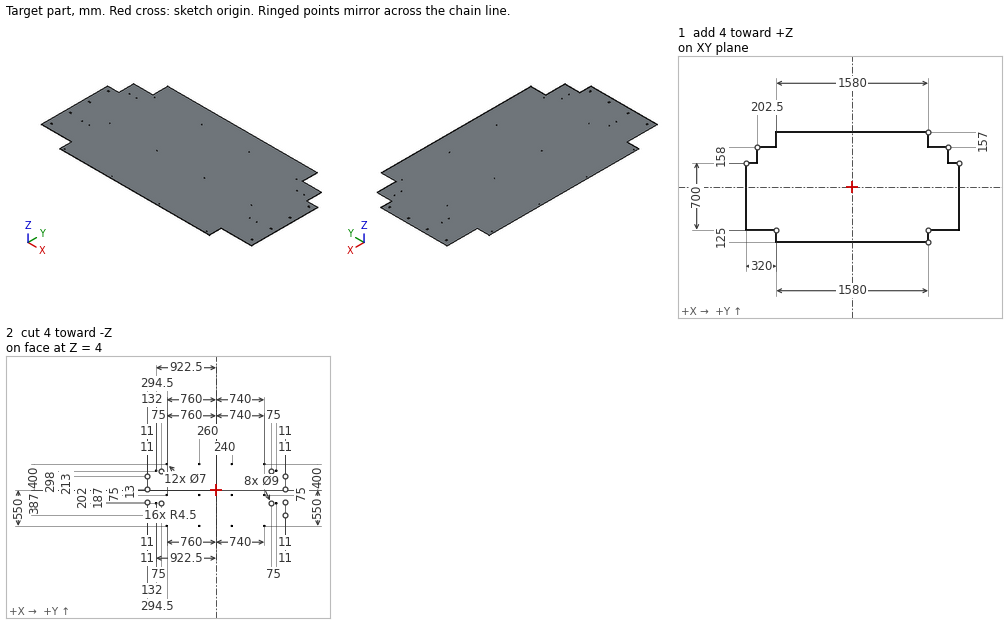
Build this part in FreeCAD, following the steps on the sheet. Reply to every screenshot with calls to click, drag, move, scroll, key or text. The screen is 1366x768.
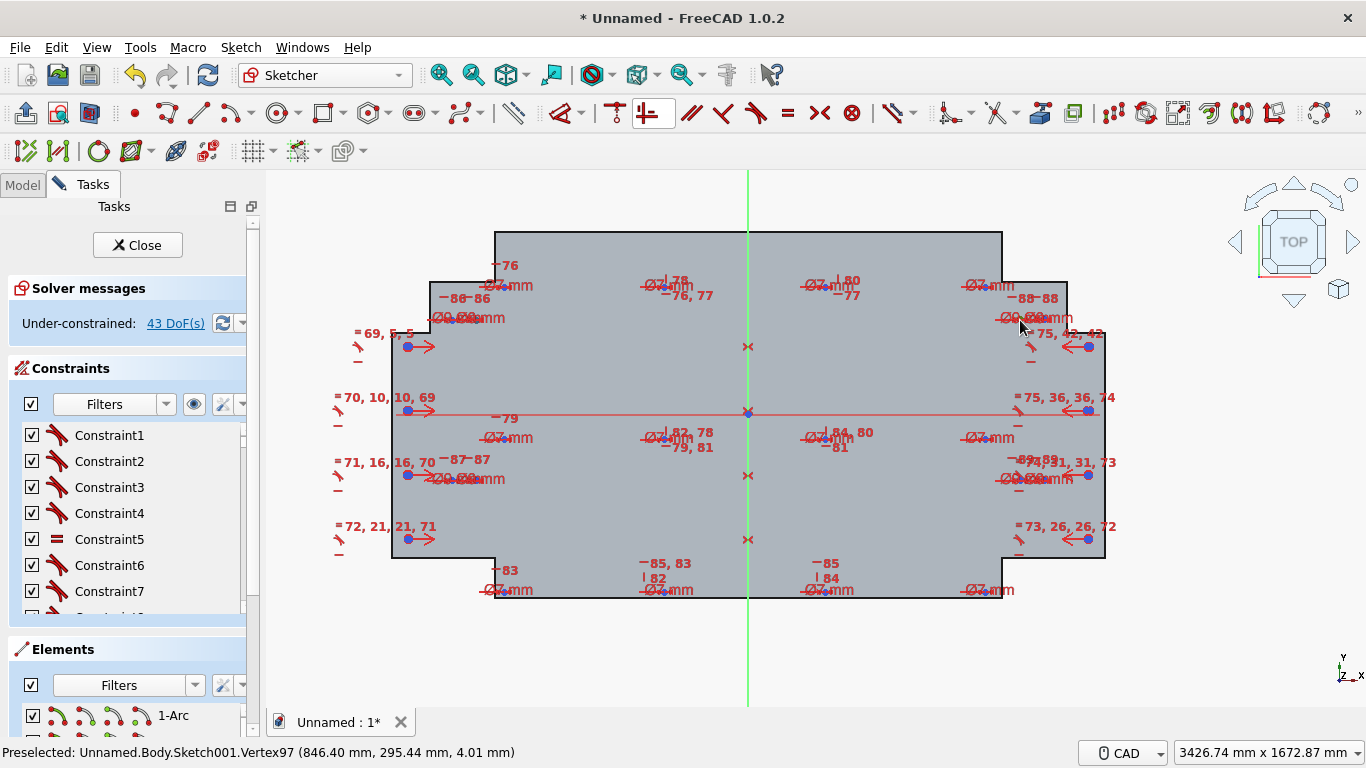
click(748, 645)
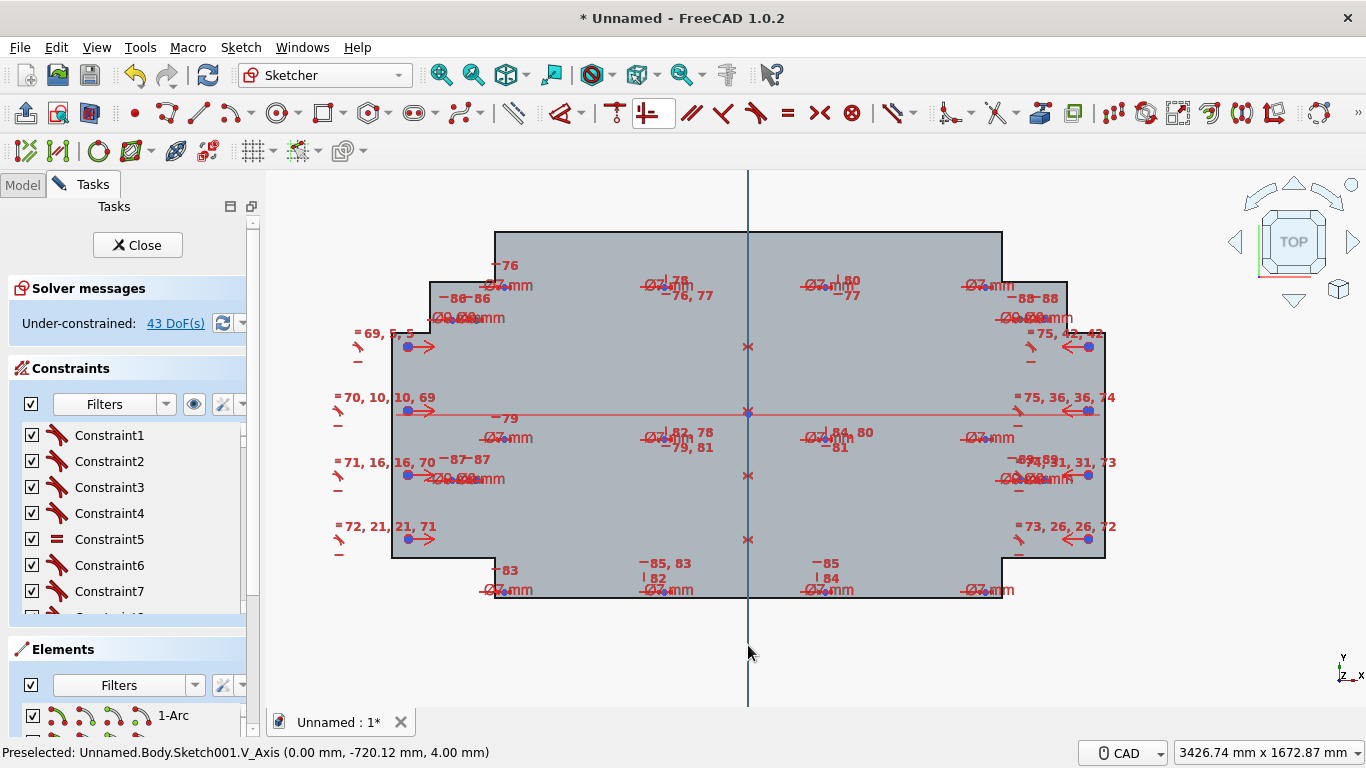
click(820, 114)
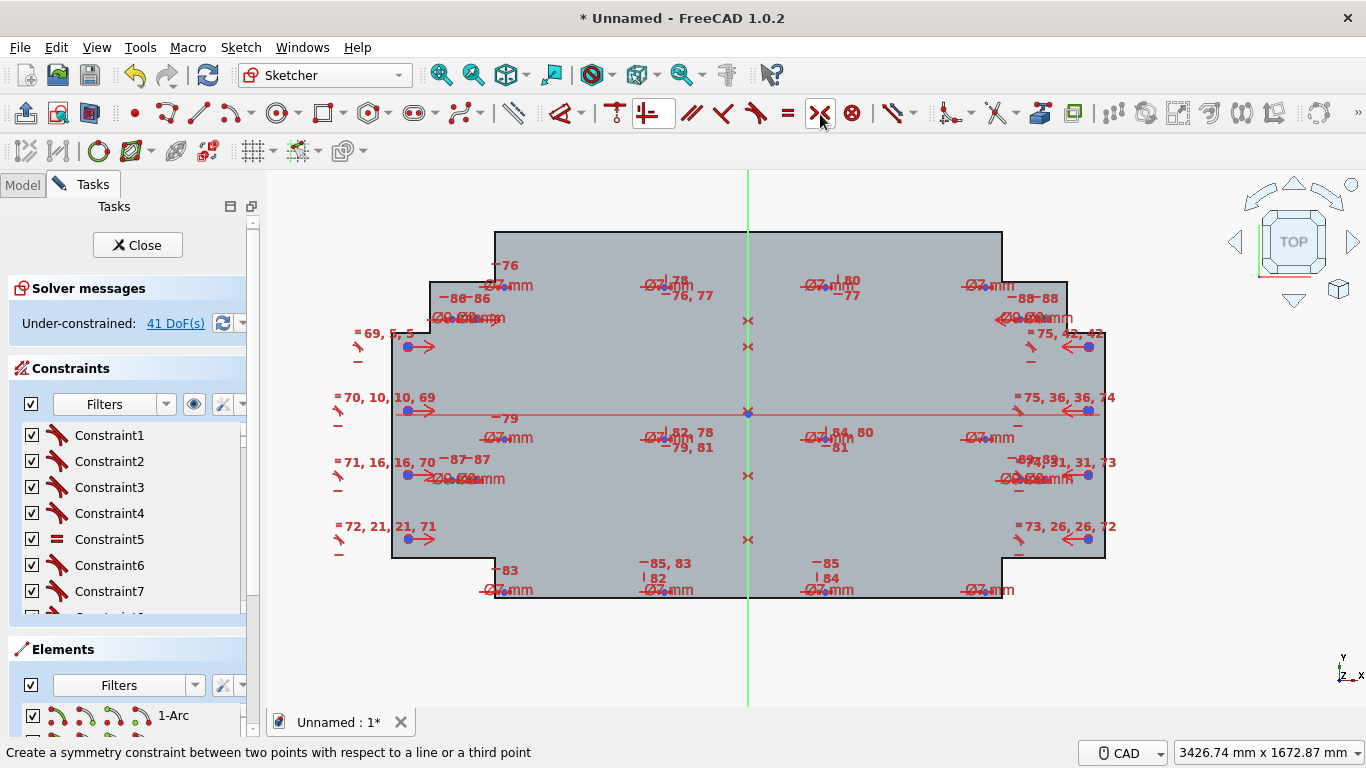
click(476, 481)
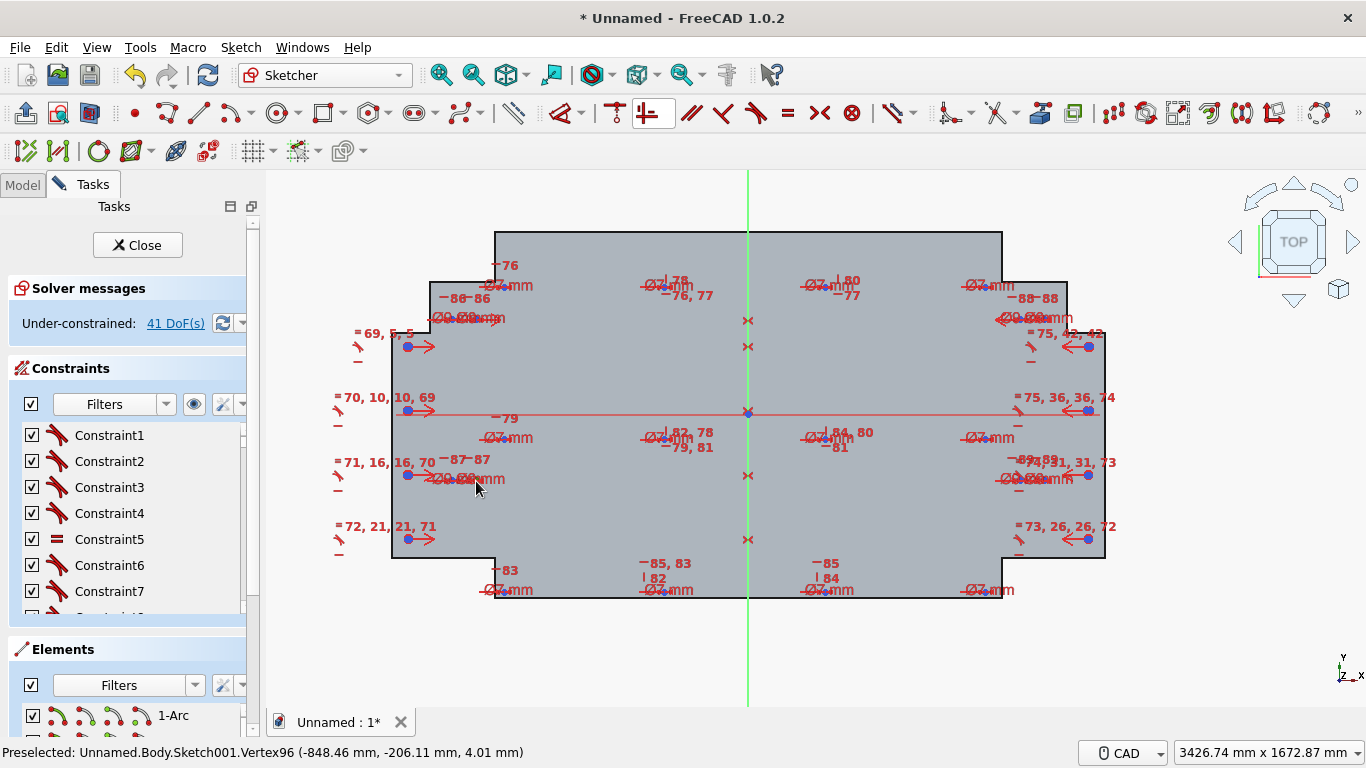
click(1020, 481)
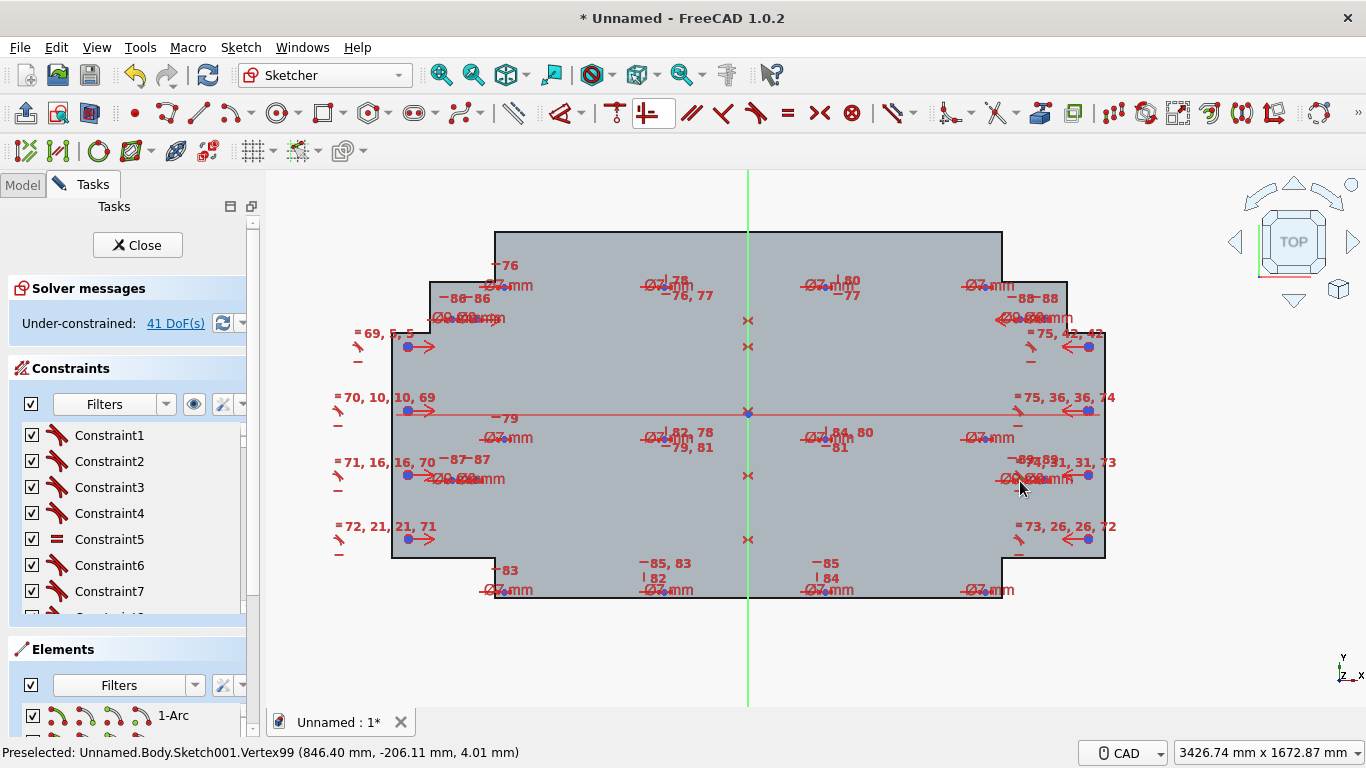
click(748, 645)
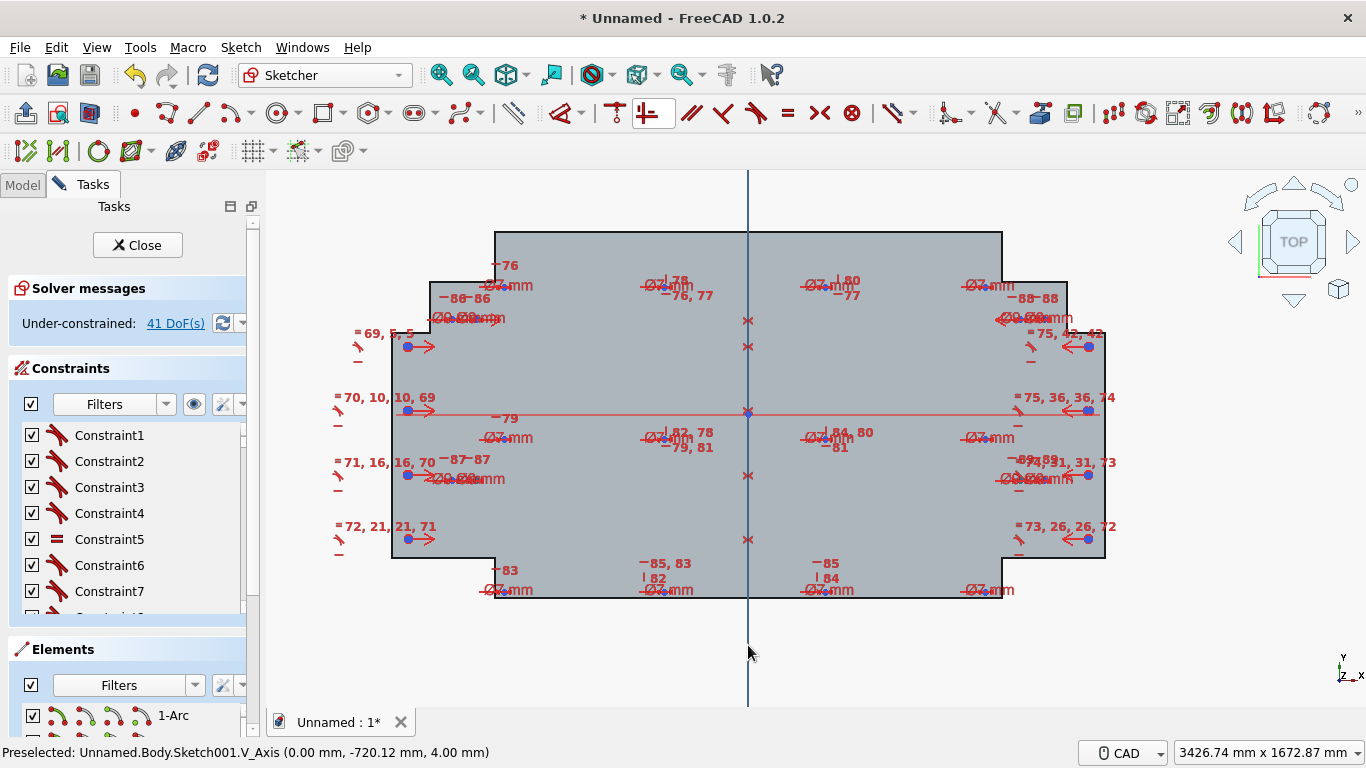
click(820, 114)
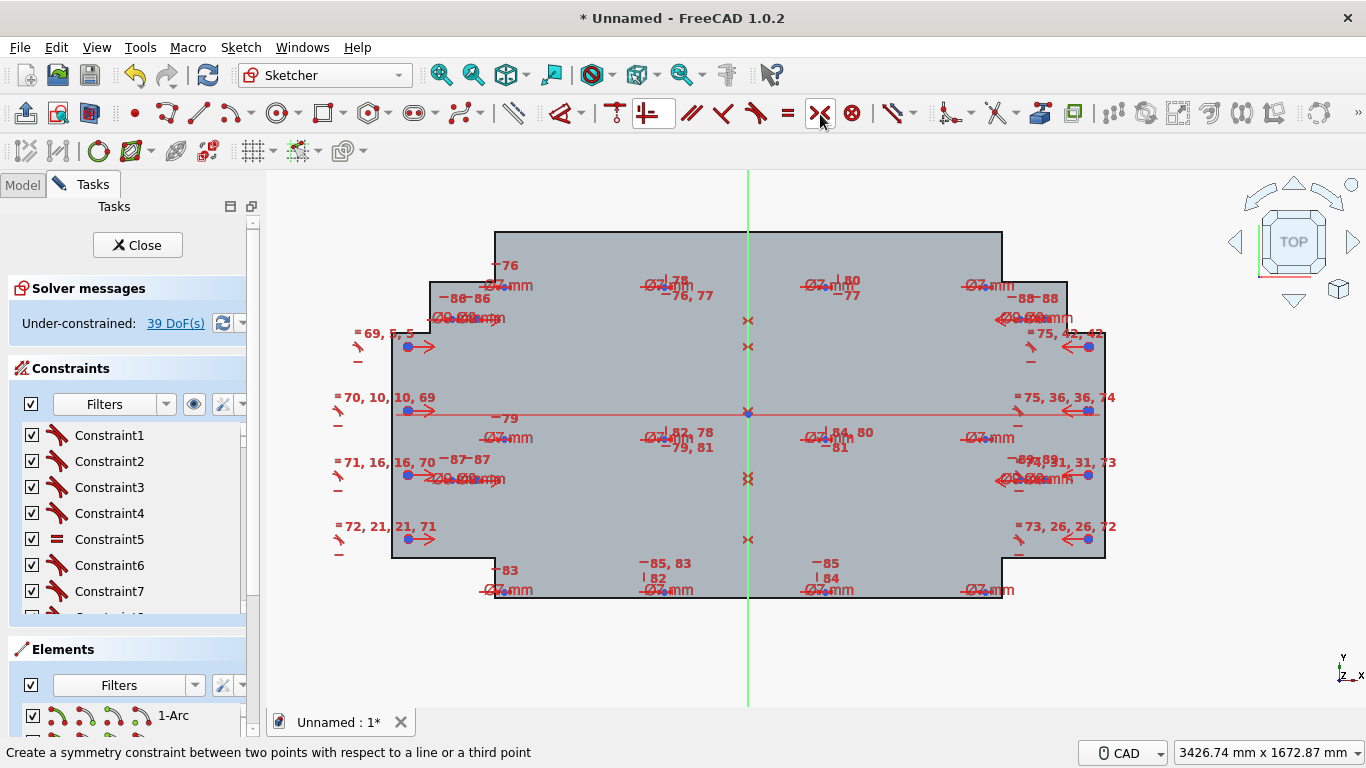
click(560, 114)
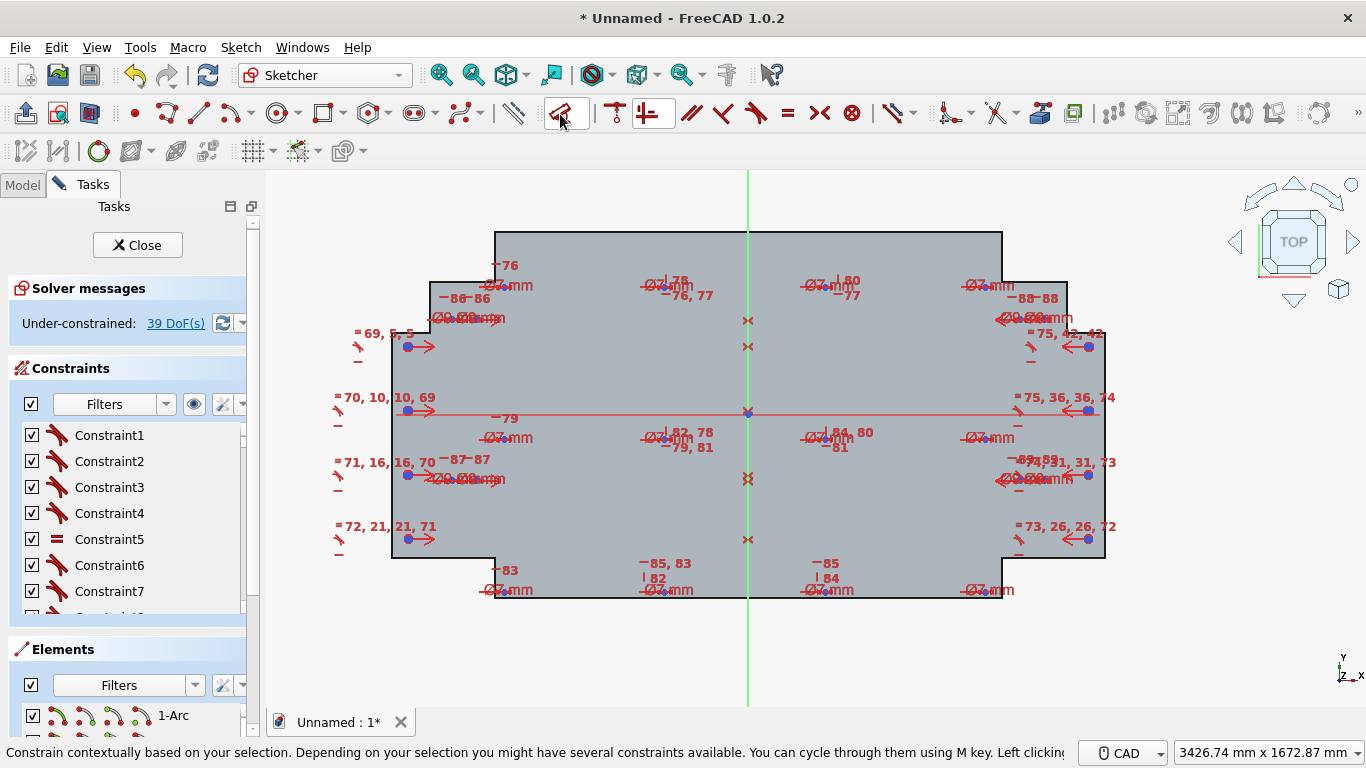
scroll(405, 347, up, 17)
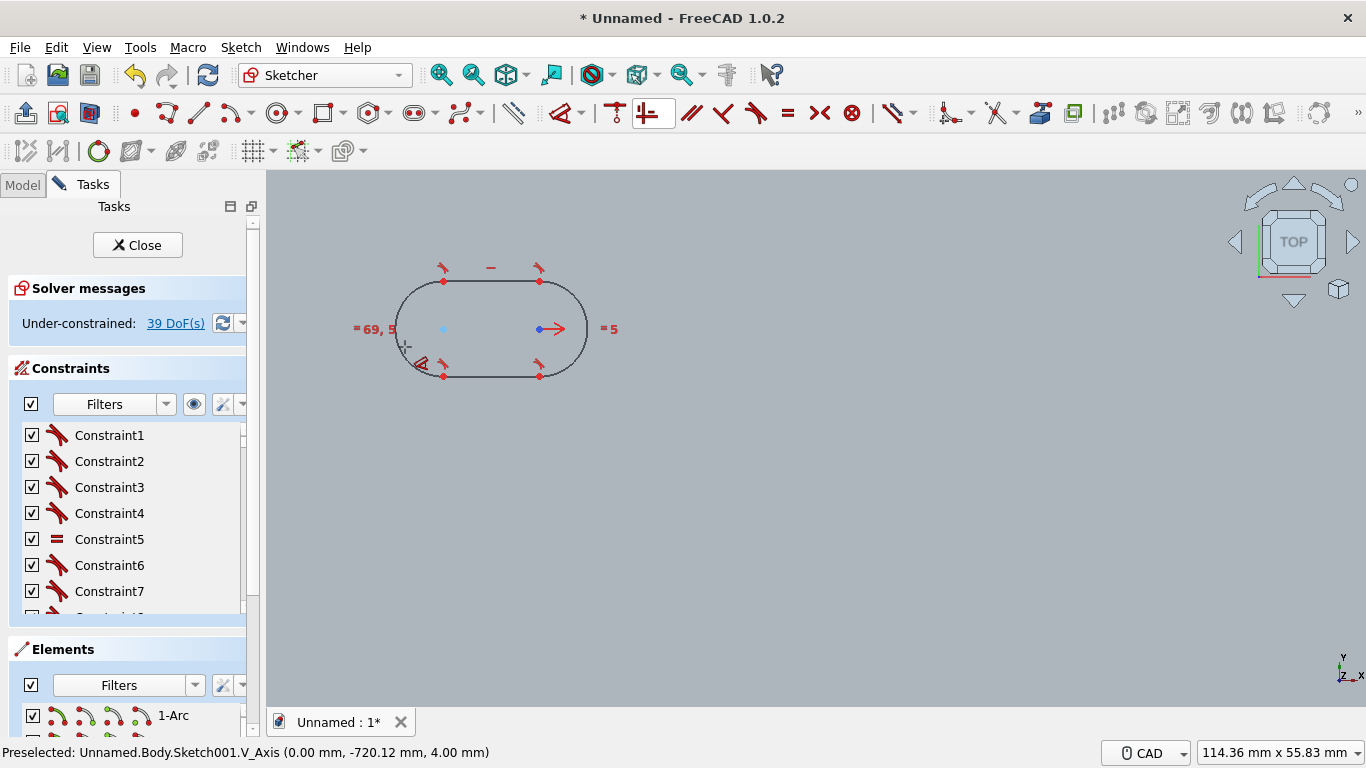
click(395, 329)
click(363, 329)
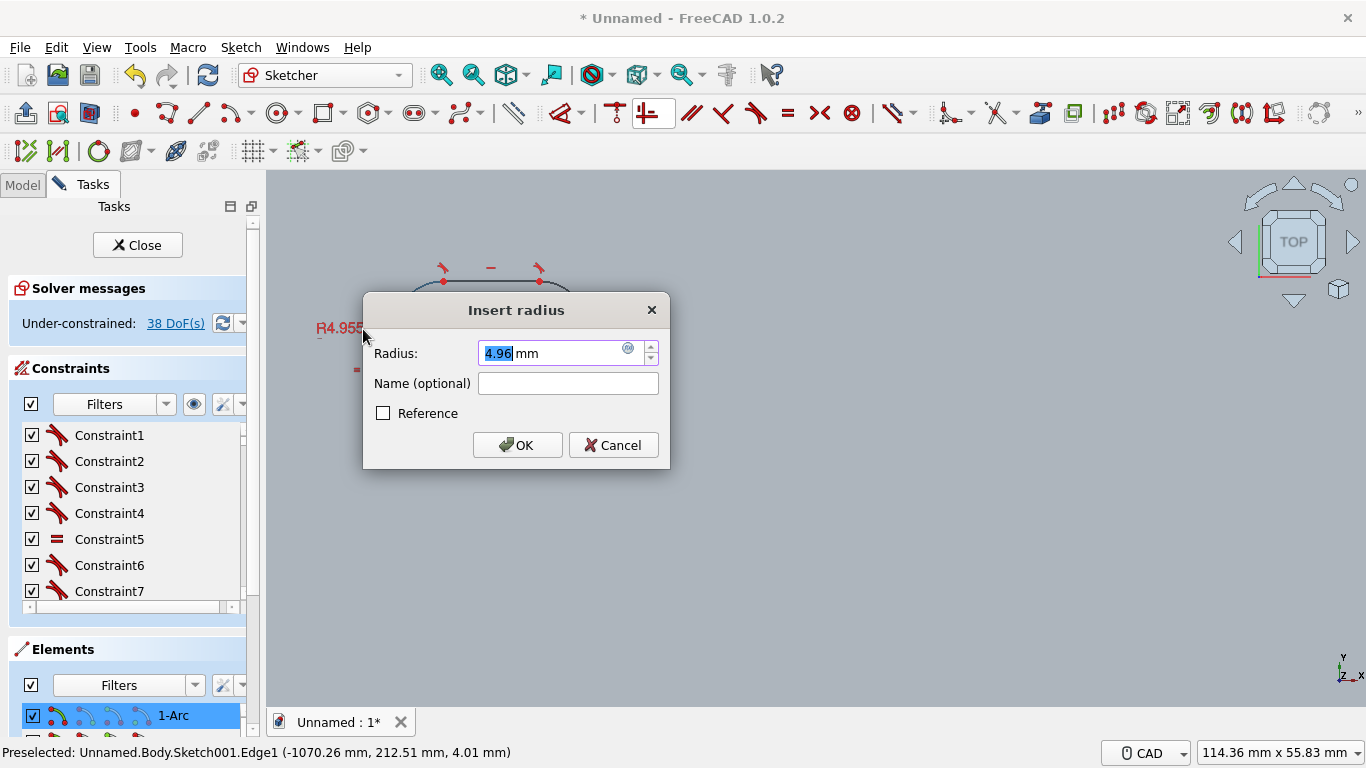
text(4.5)
key(Return)